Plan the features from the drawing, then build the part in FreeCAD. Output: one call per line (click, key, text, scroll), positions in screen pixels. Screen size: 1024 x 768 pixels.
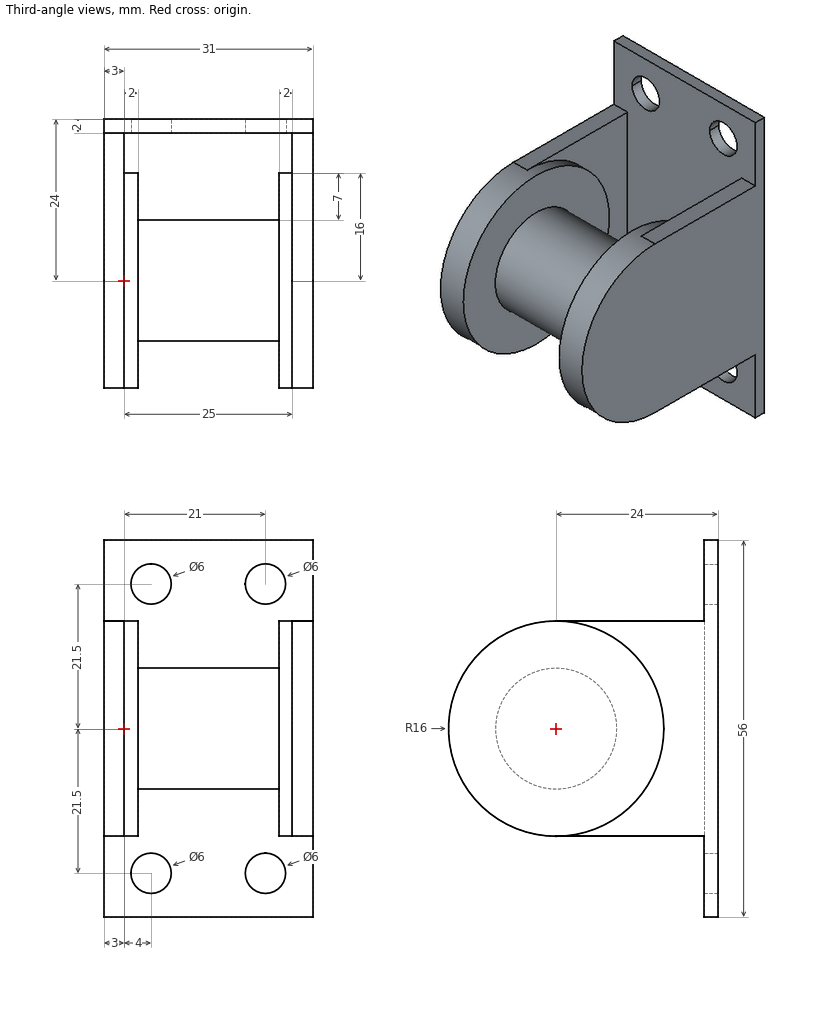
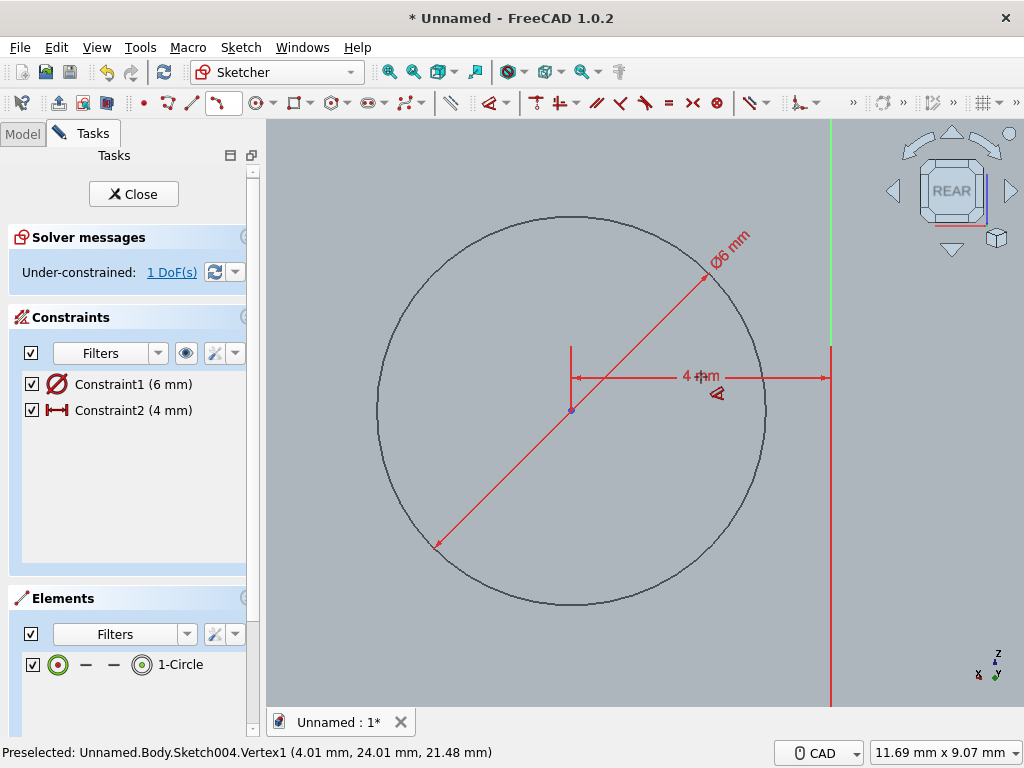
click(571, 411)
click(537, 545)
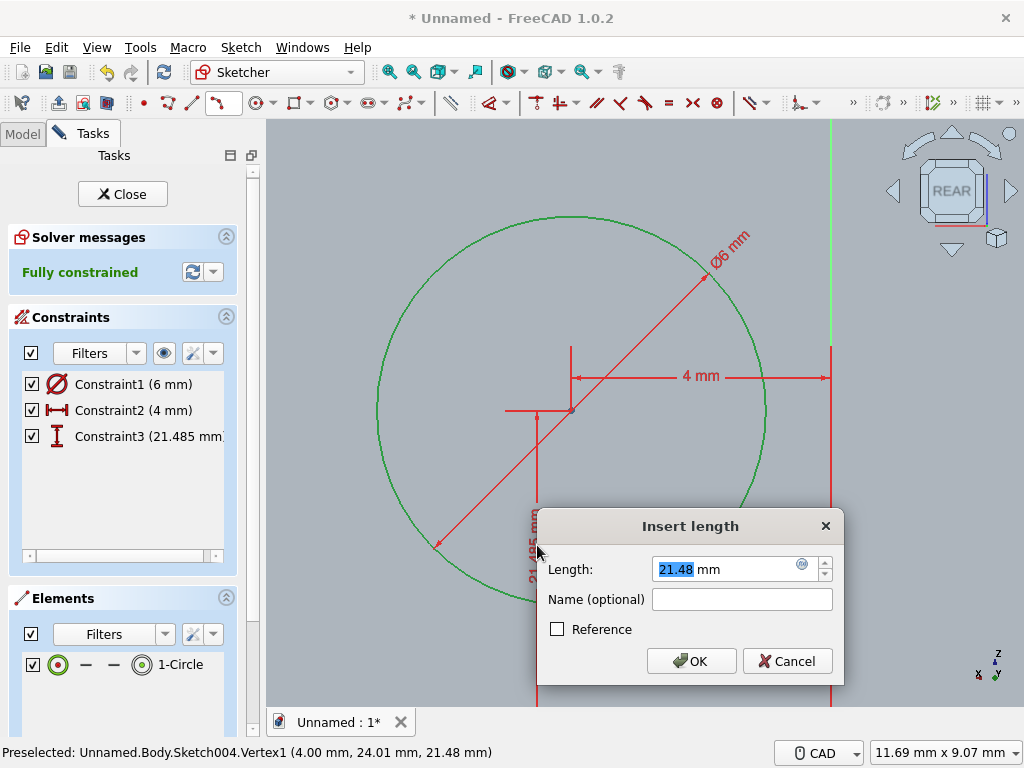
text(21.5)
key(Return)
key(Escape)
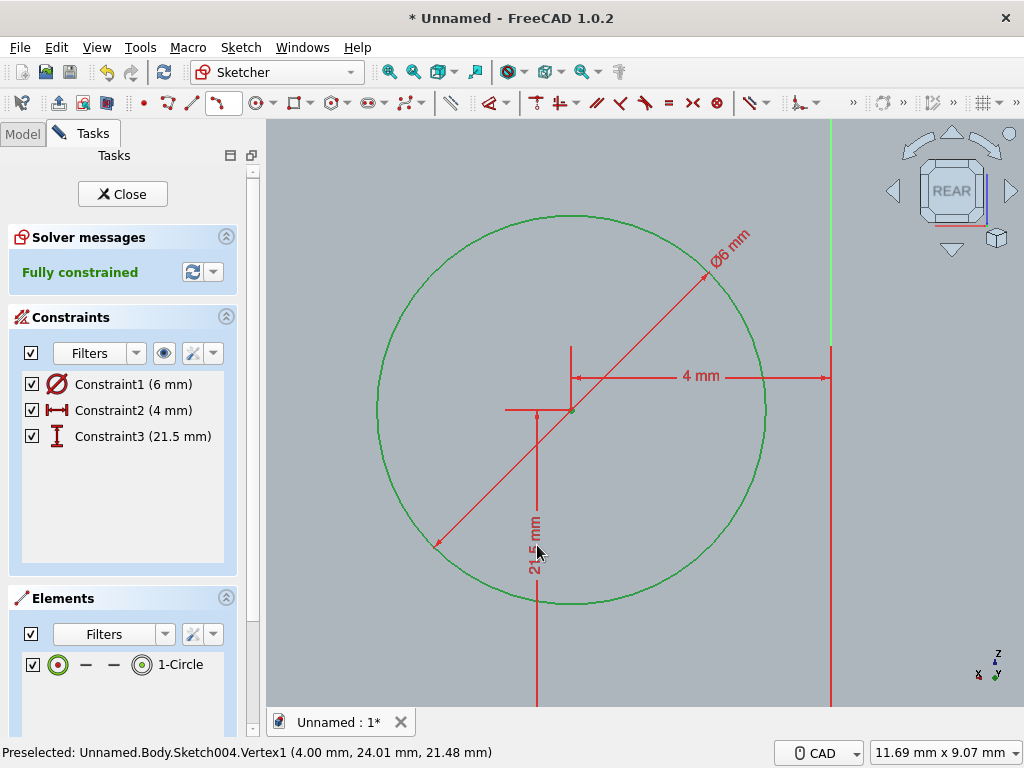
click(123, 194)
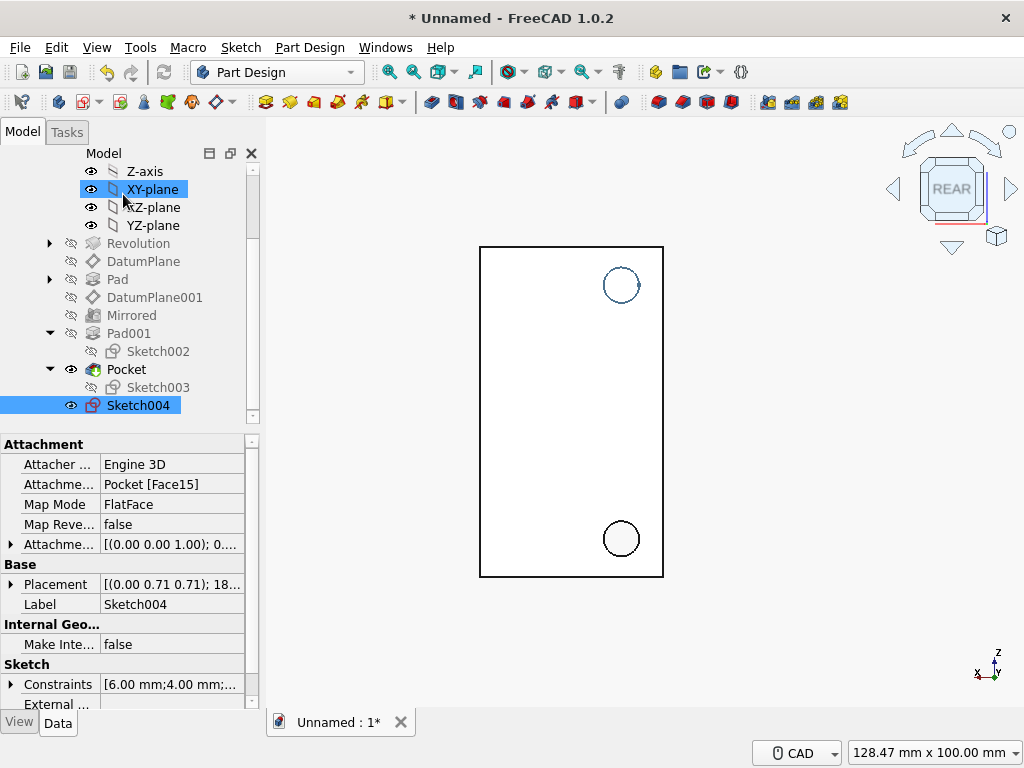
click(432, 102)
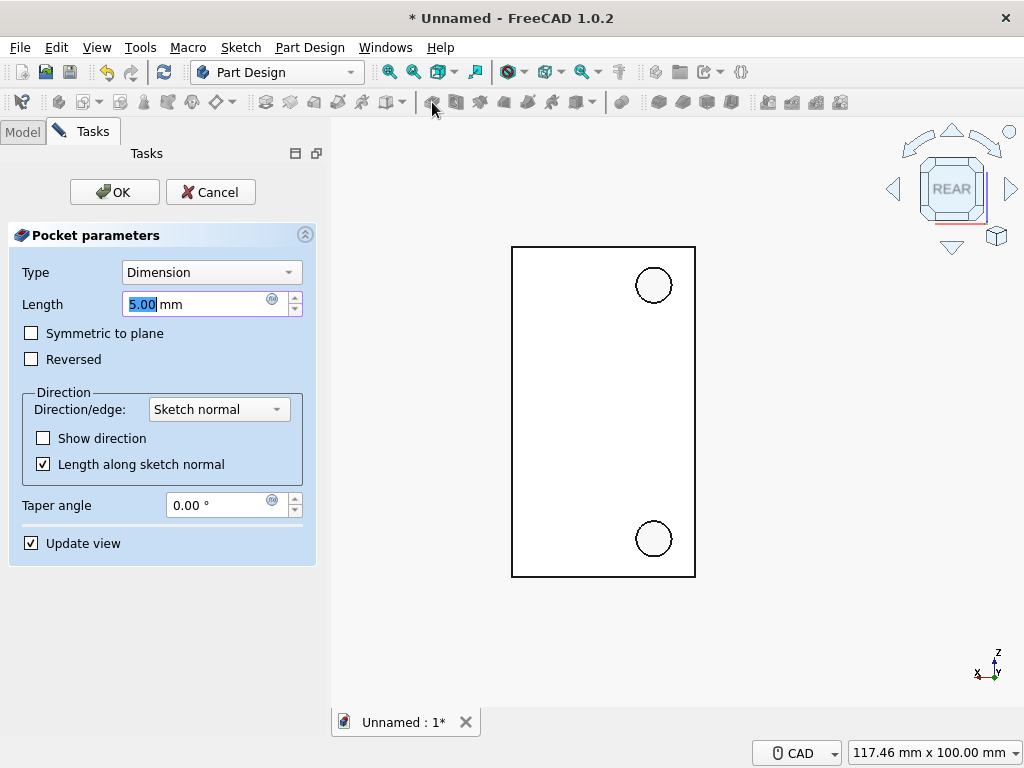
click(212, 272)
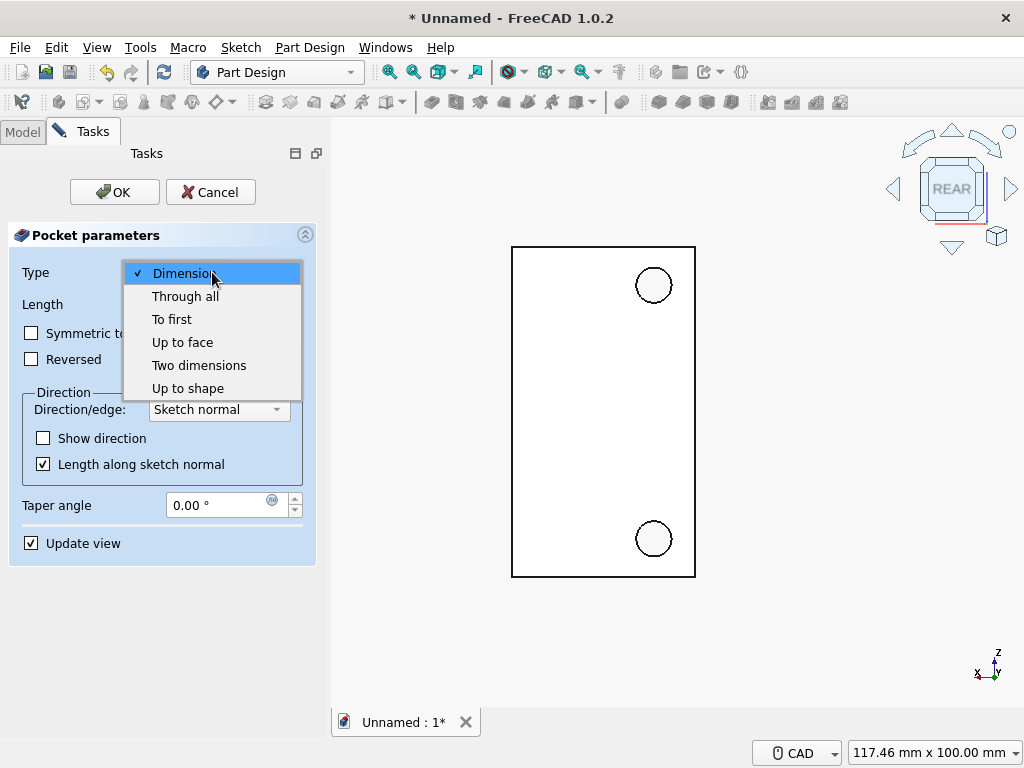
click(212, 320)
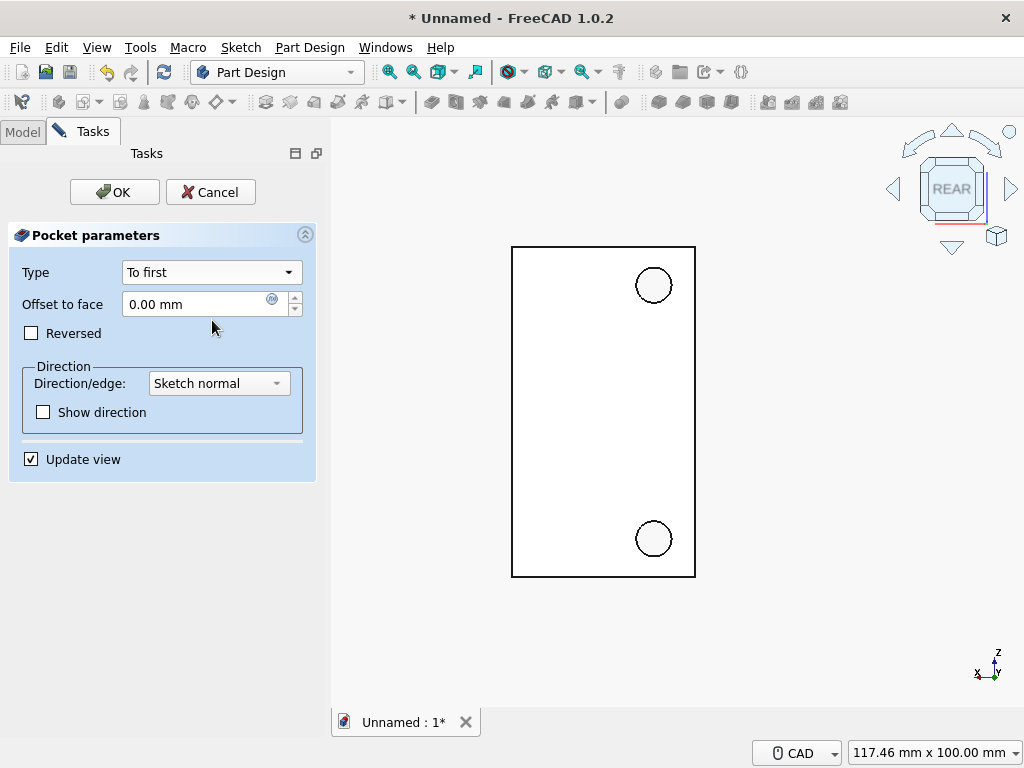
click(115, 192)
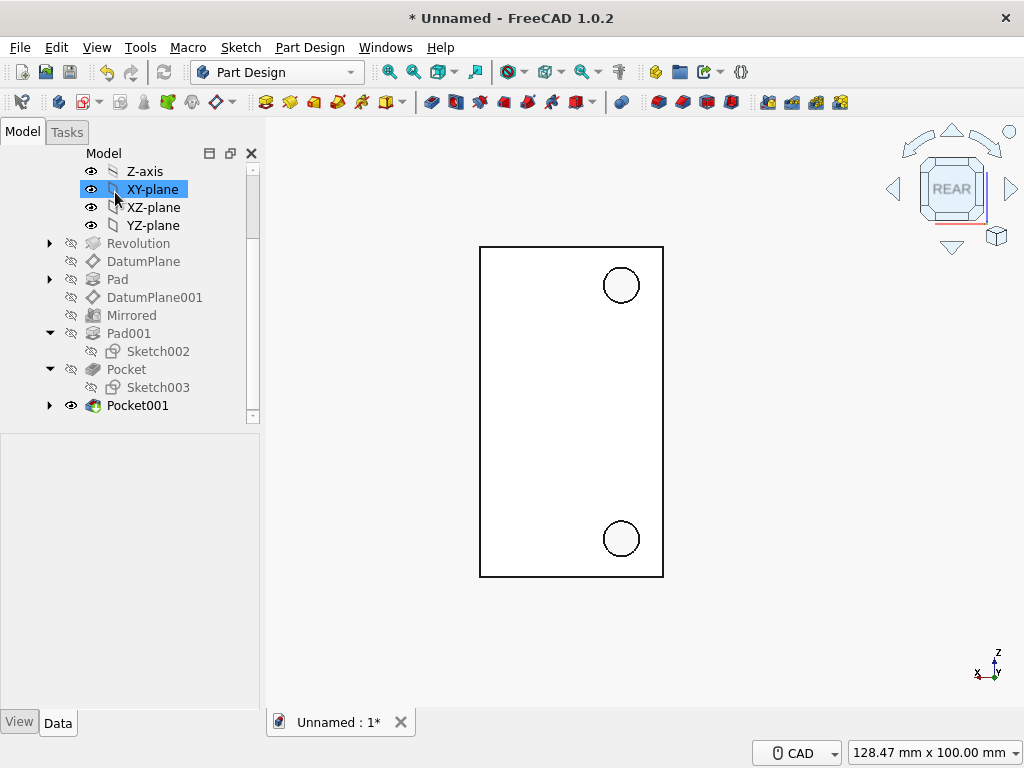
click(571, 411)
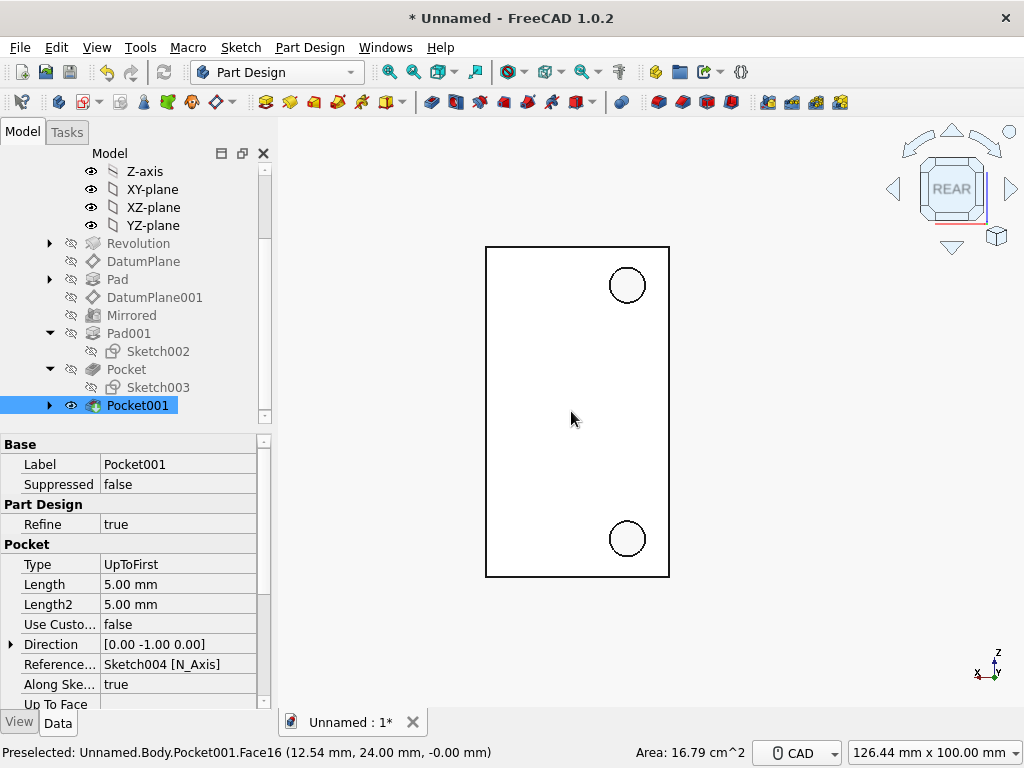
click(84, 102)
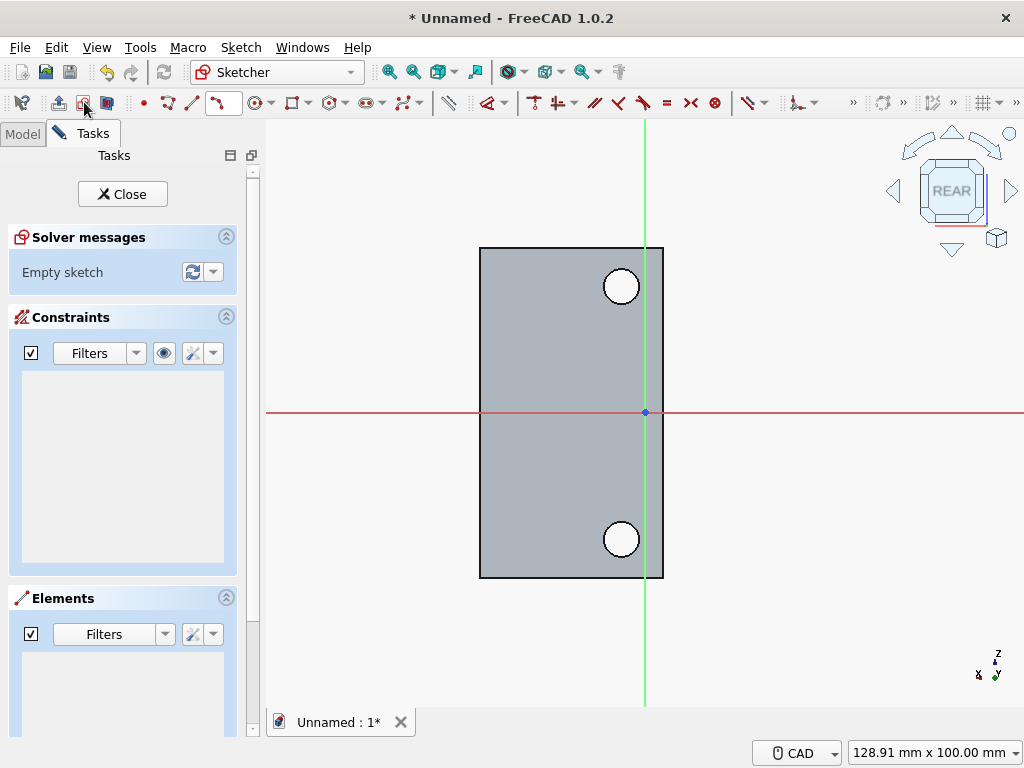
scroll(516, 274, up, 12)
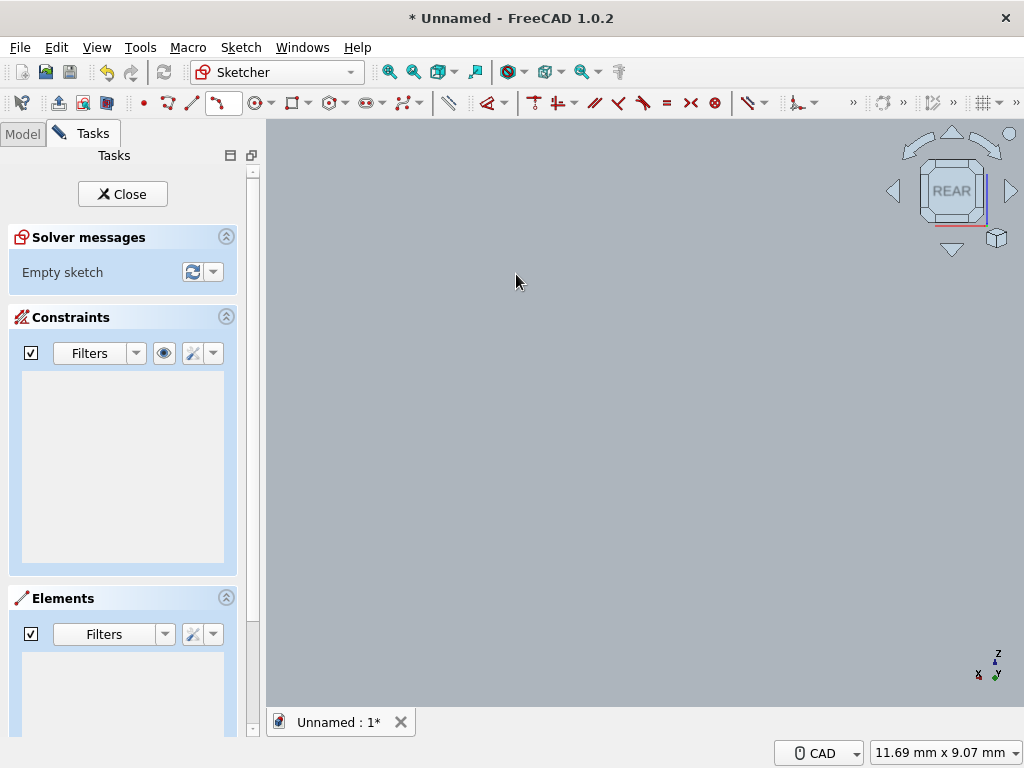
click(256, 104)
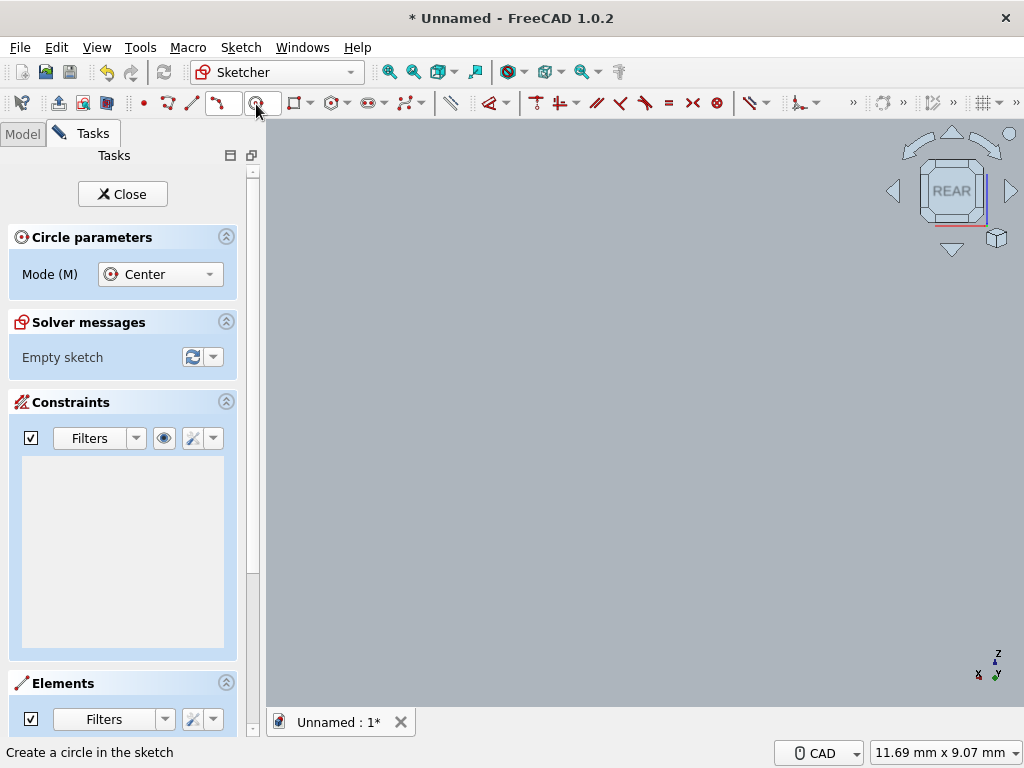
click(574, 410)
click(711, 273)
key(Escape)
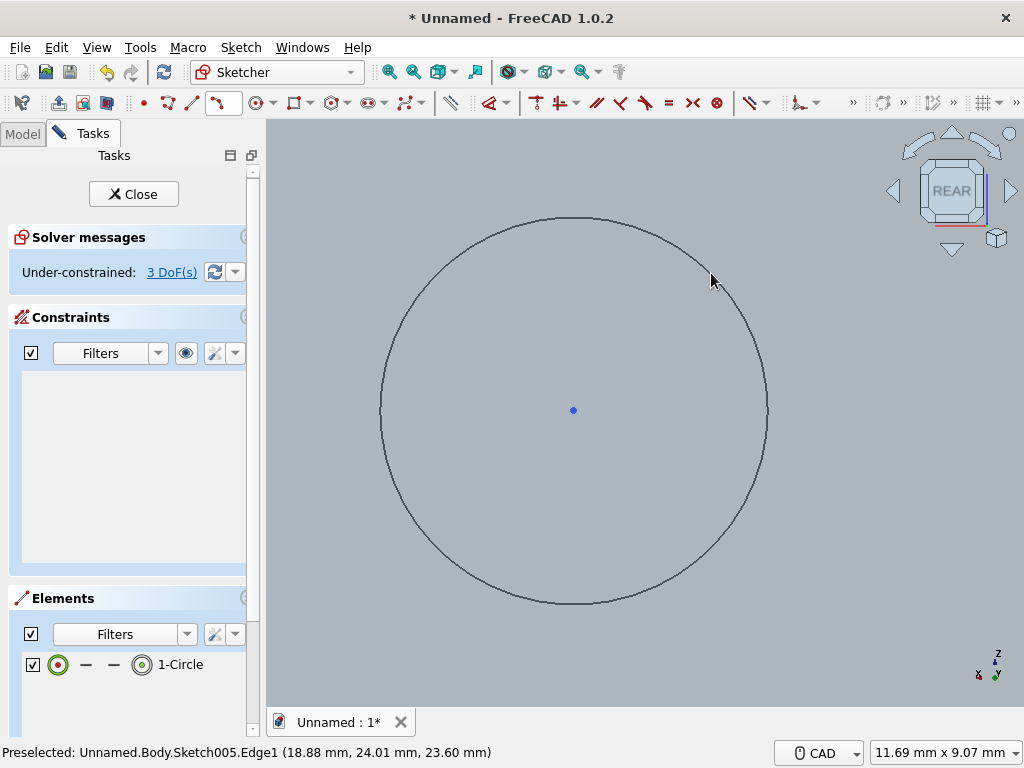
click(490, 104)